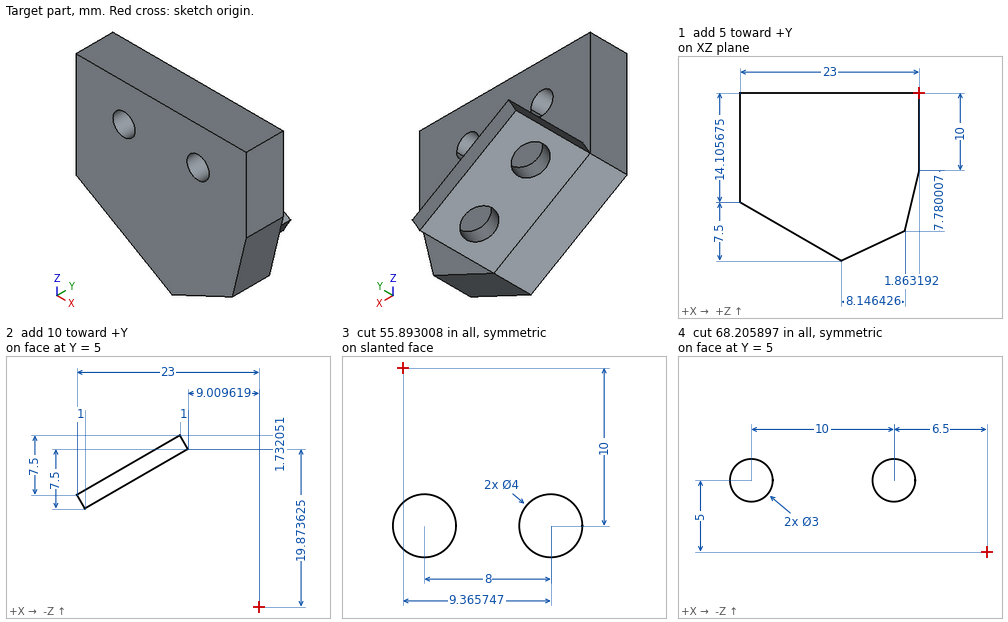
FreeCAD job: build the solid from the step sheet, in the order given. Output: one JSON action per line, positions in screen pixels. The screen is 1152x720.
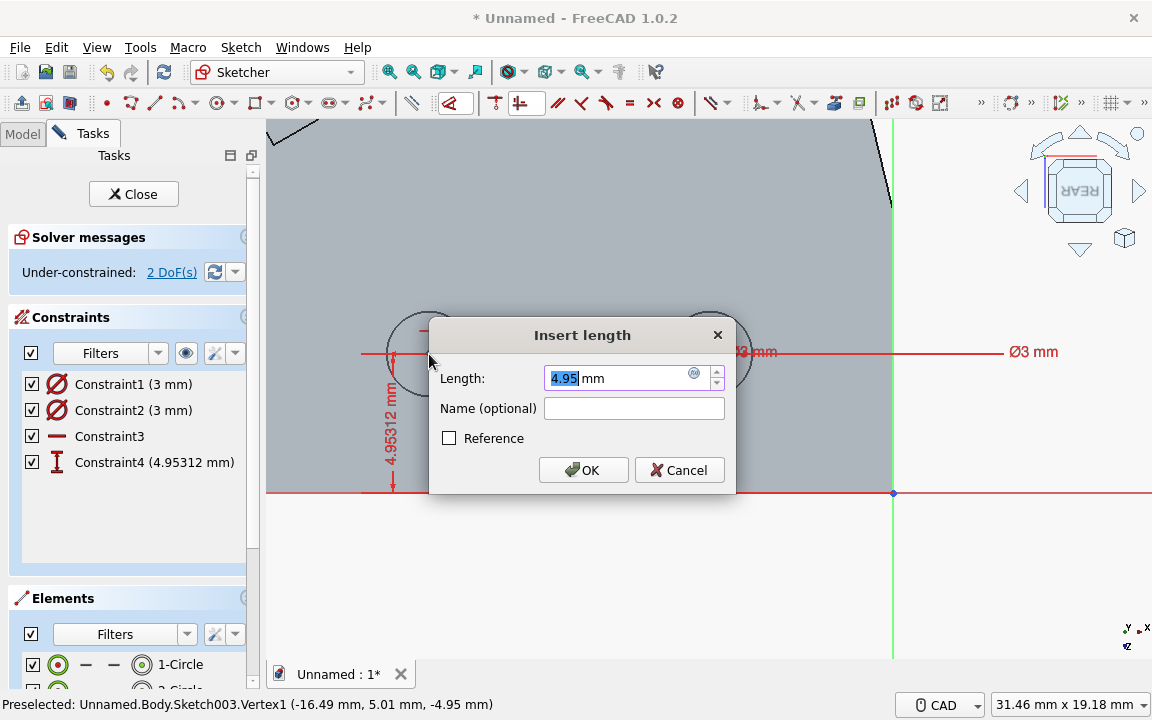
{"action": "type", "text": "5"}
{"action": "key", "text": "Return"}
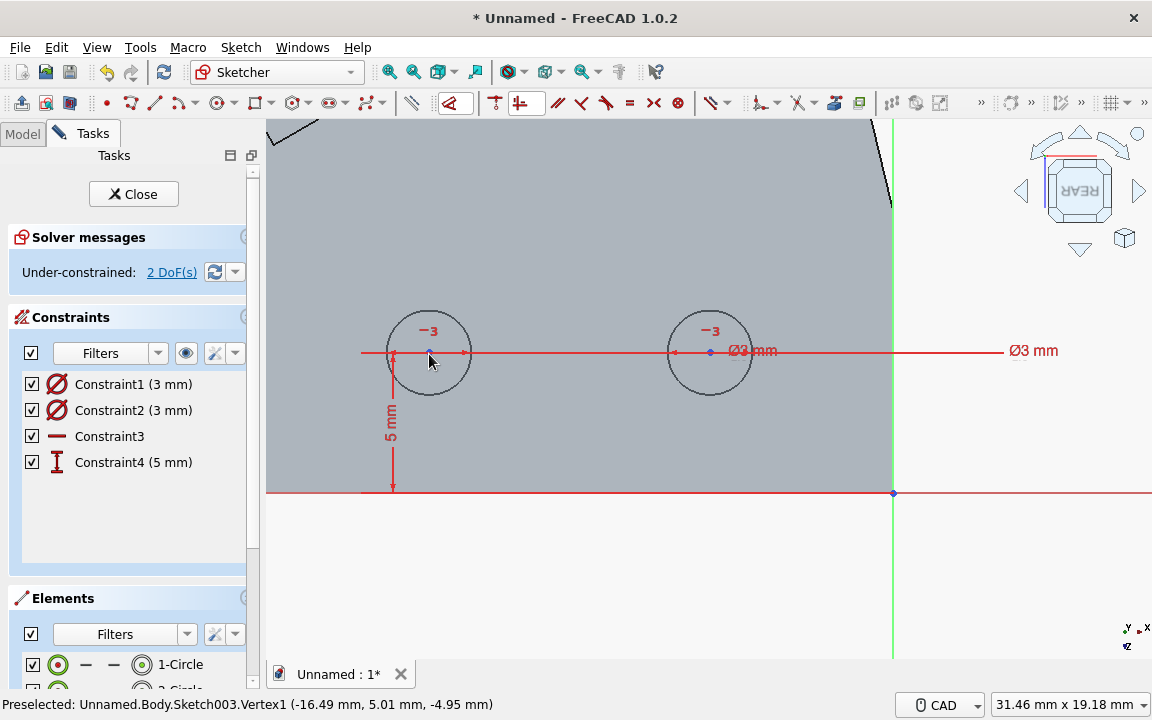
{"action": "left_click", "coordinate": [710, 353]}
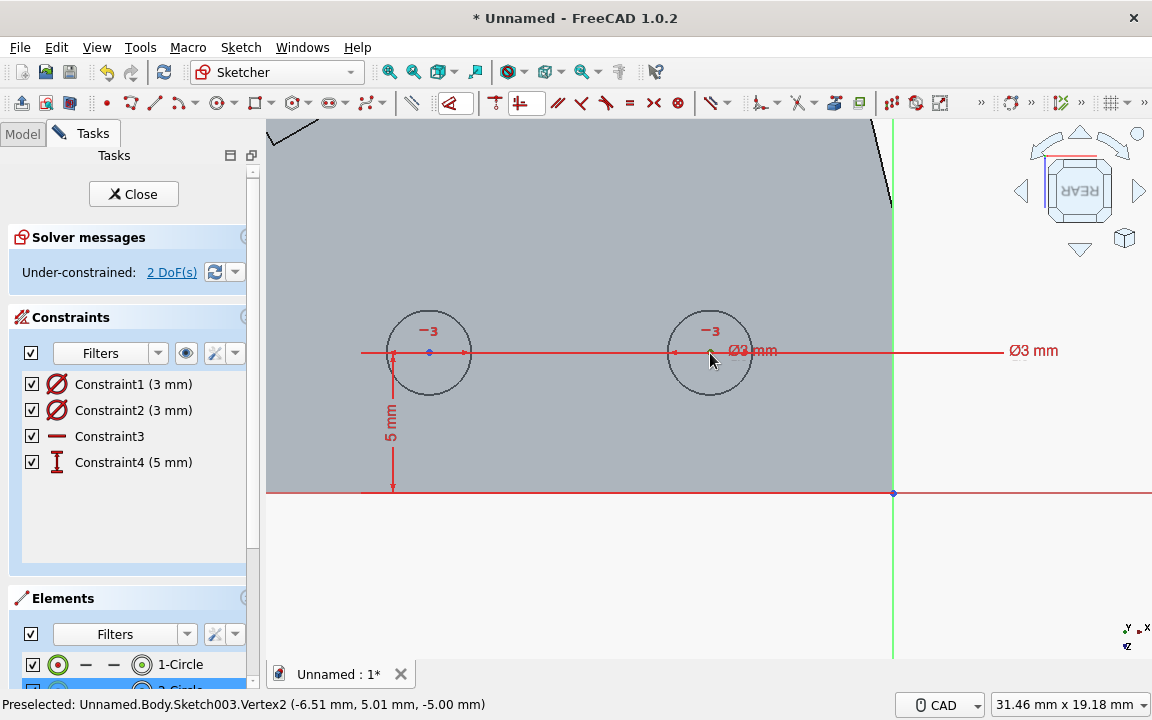
{"action": "left_click", "coordinate": [468, 104]}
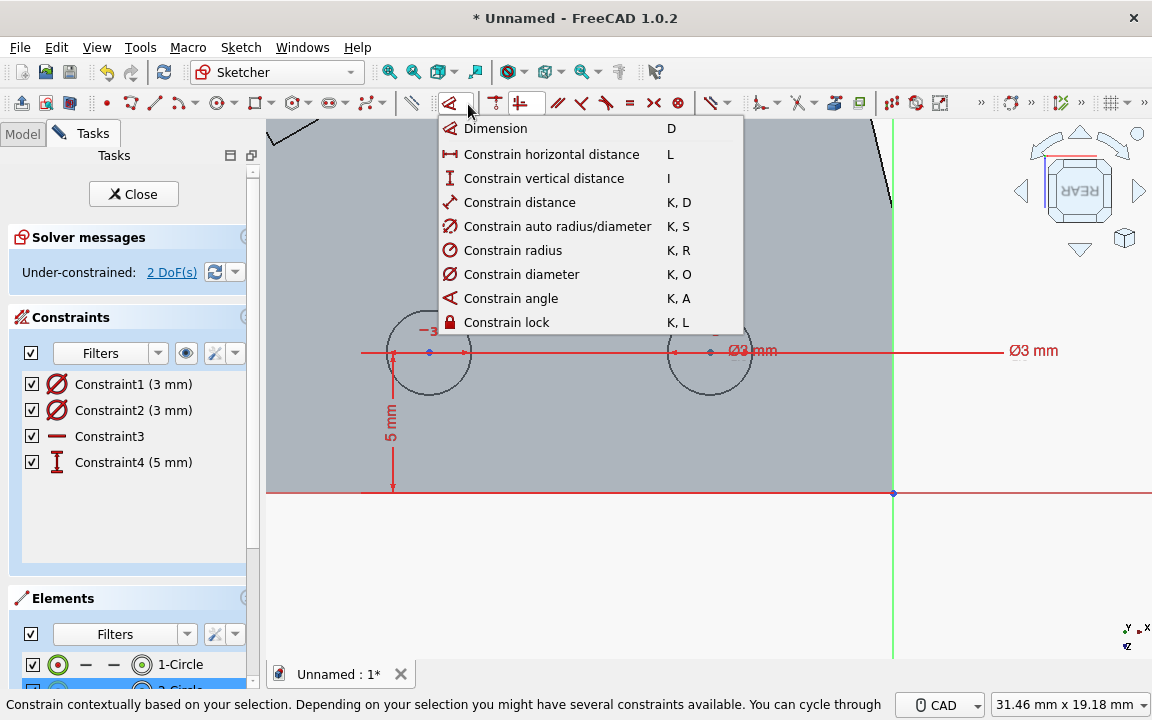
{"action": "left_click", "coordinate": [591, 154]}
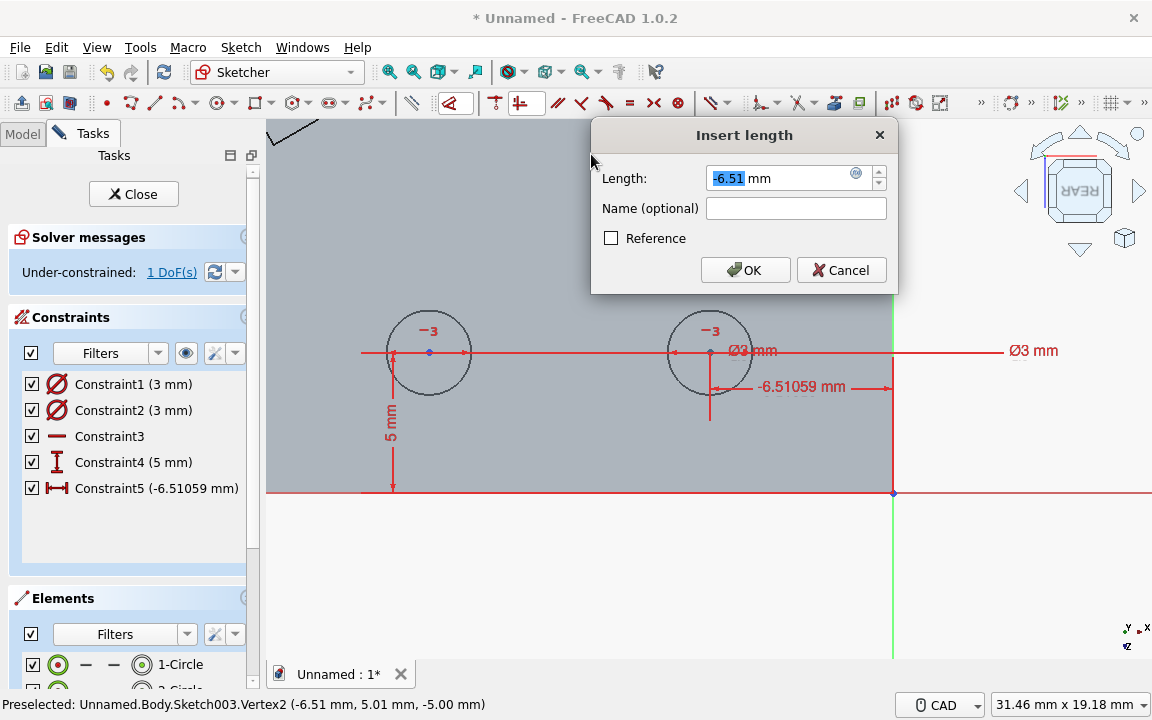
{"action": "type", "text": "-6.5"}
{"action": "key", "text": "Return"}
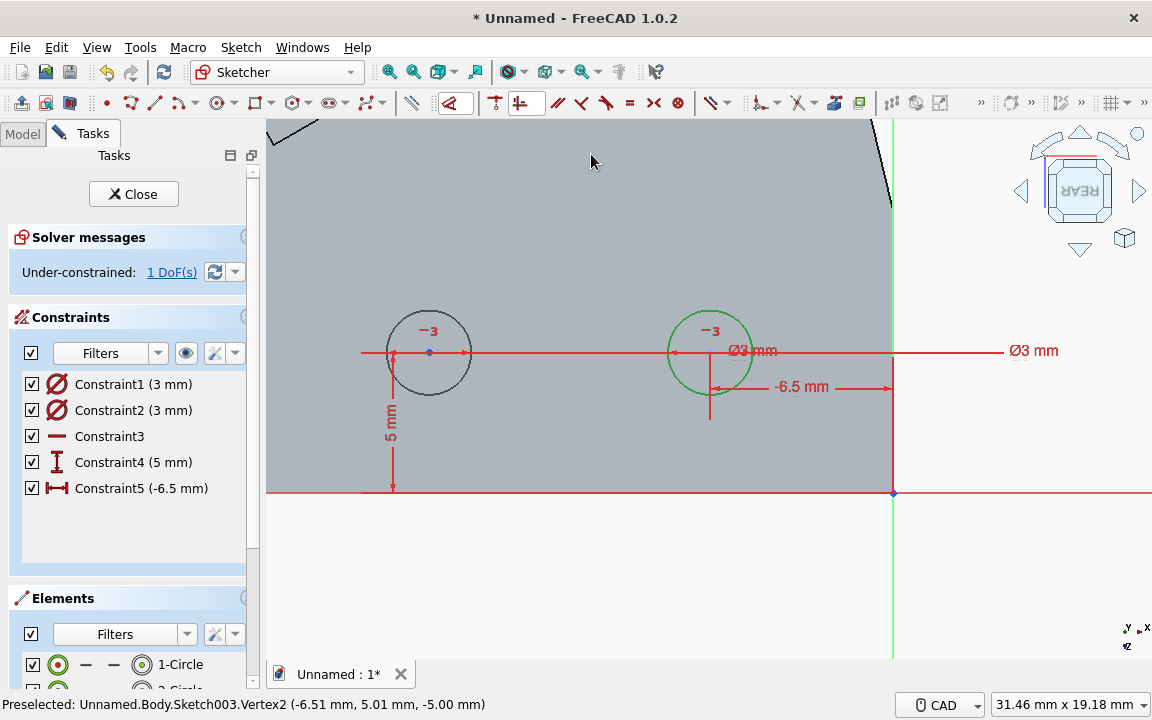
{"action": "left_click", "coordinate": [429, 353]}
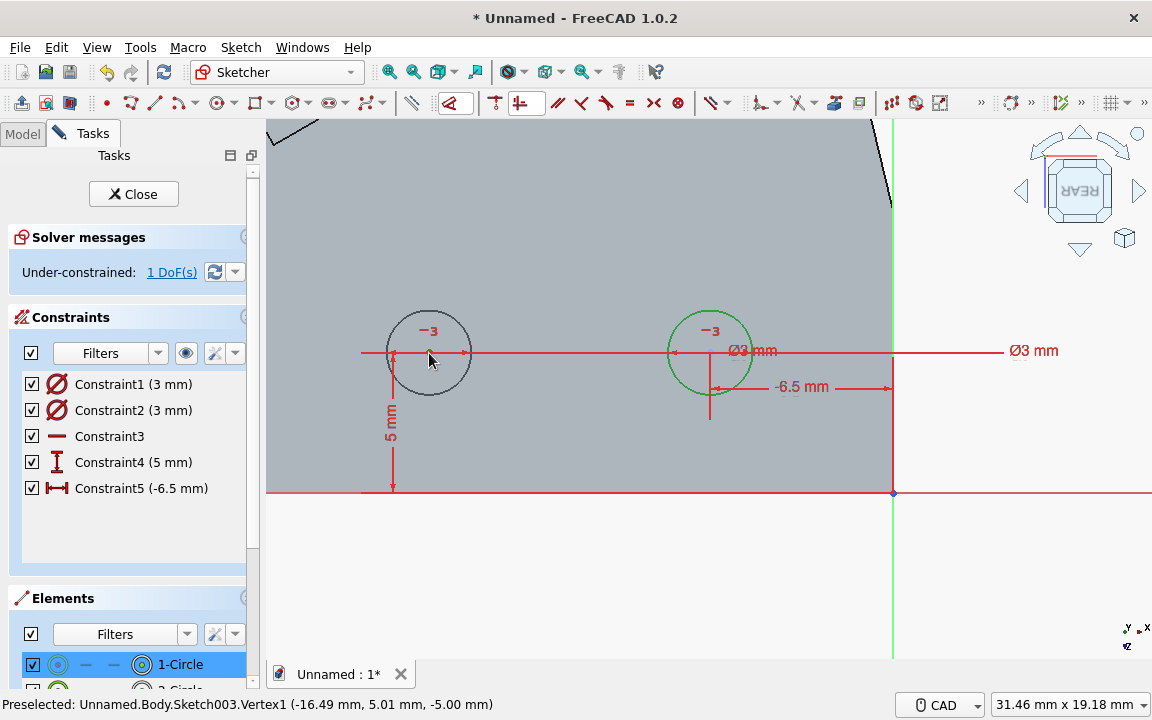
{"action": "left_click", "coordinate": [710, 353]}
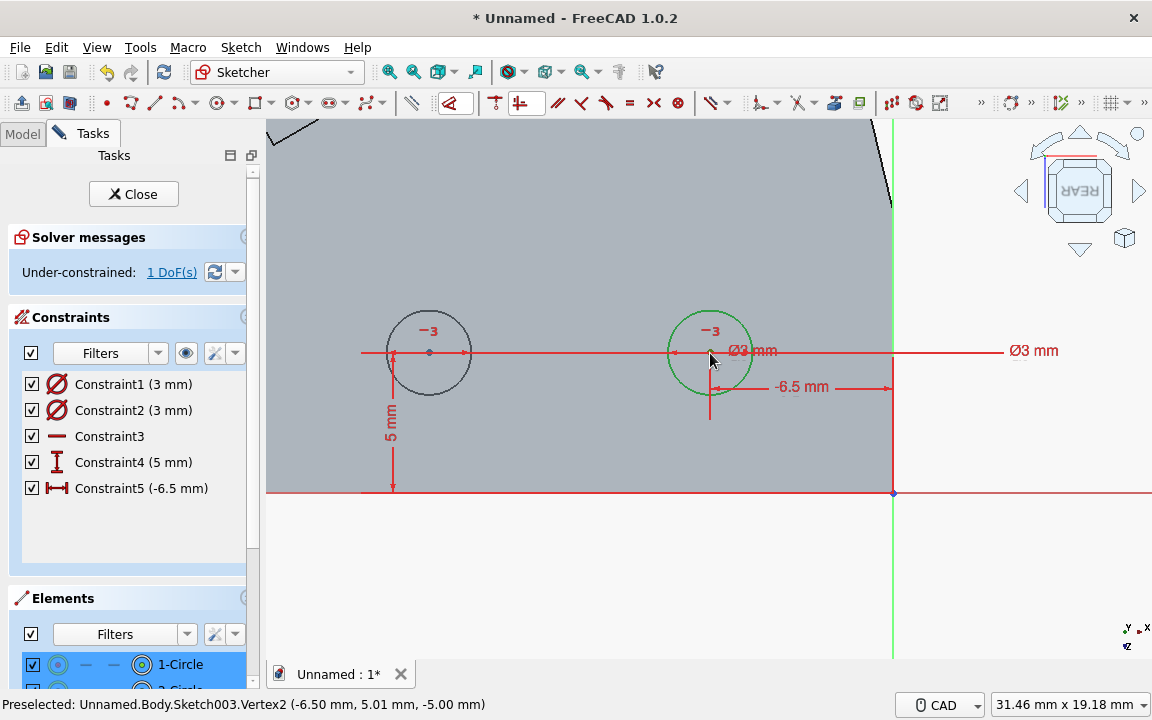
{"action": "key", "text": "l"}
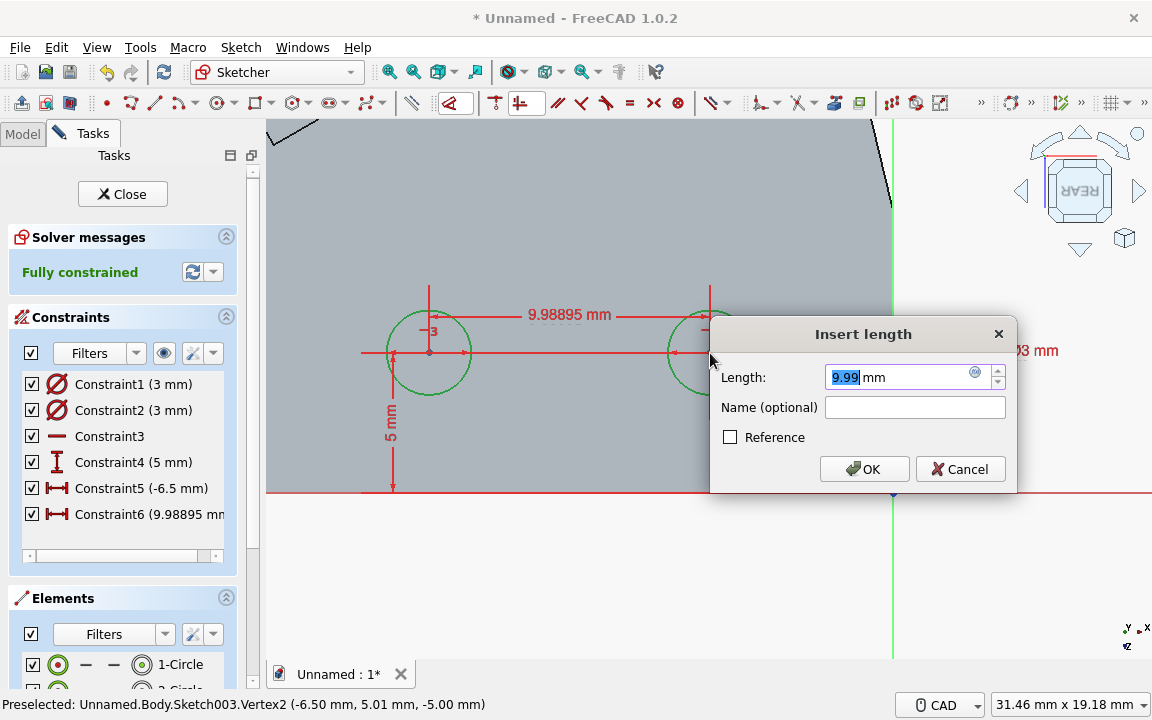
{"action": "type", "text": "10"}
{"action": "key", "text": "Return"}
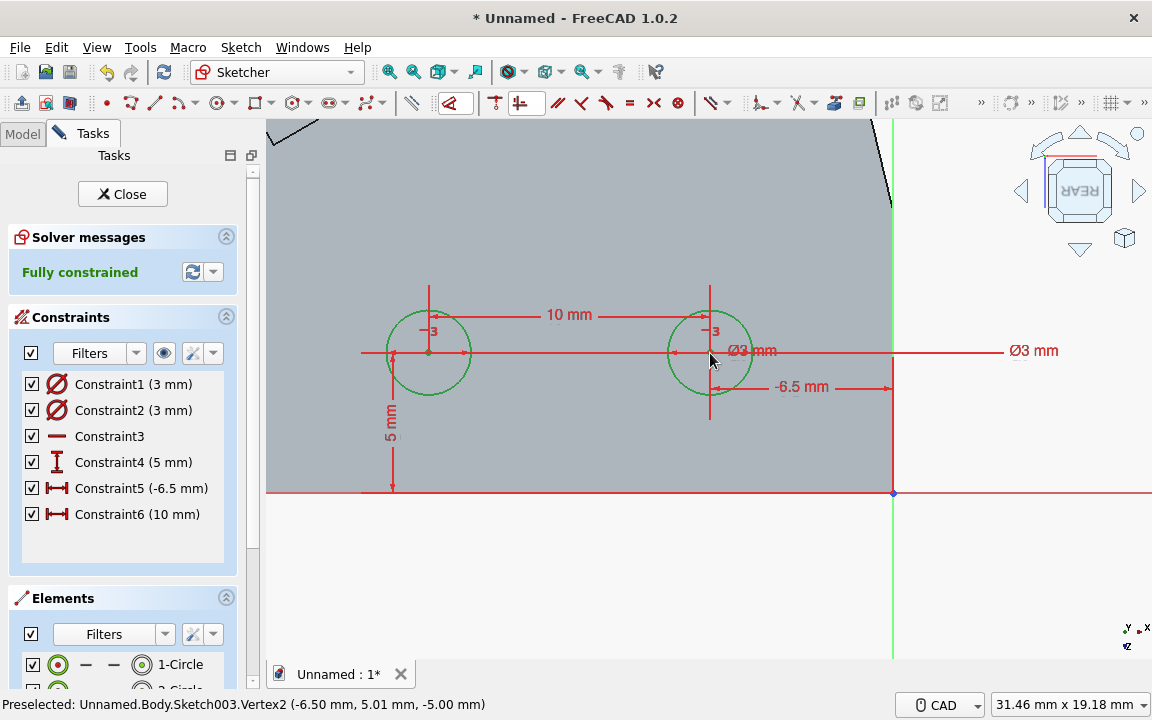
{"action": "left_click", "coordinate": [123, 194]}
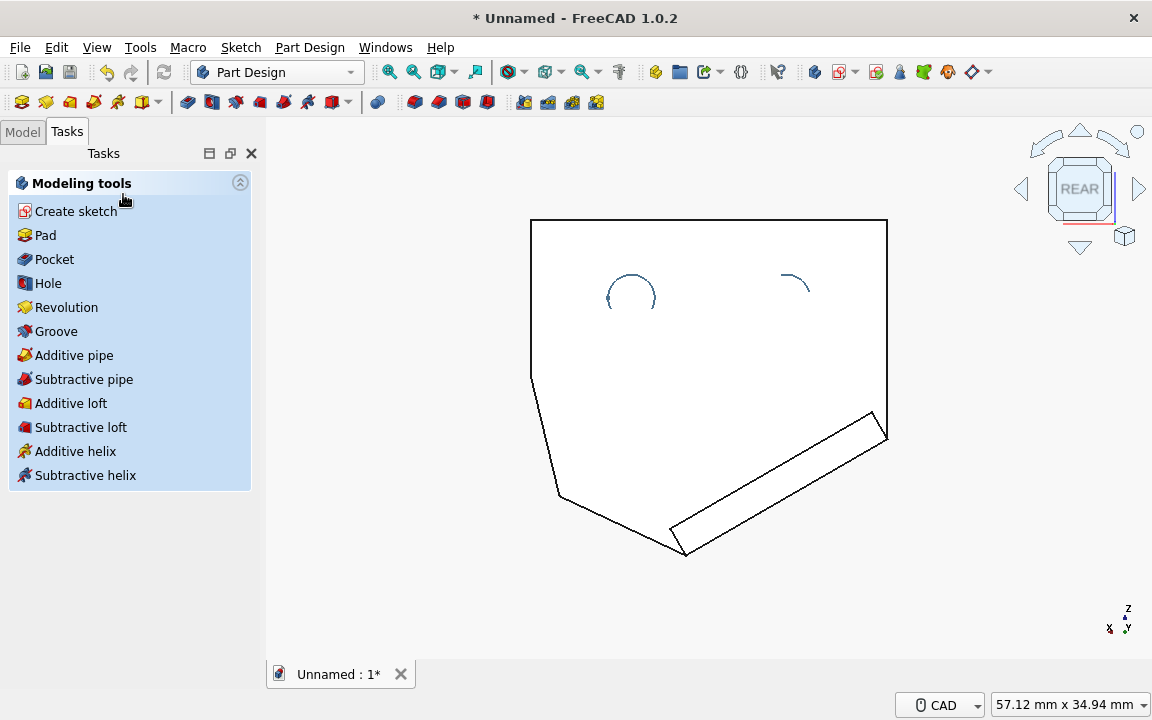
{"action": "left_click", "coordinate": [188, 102]}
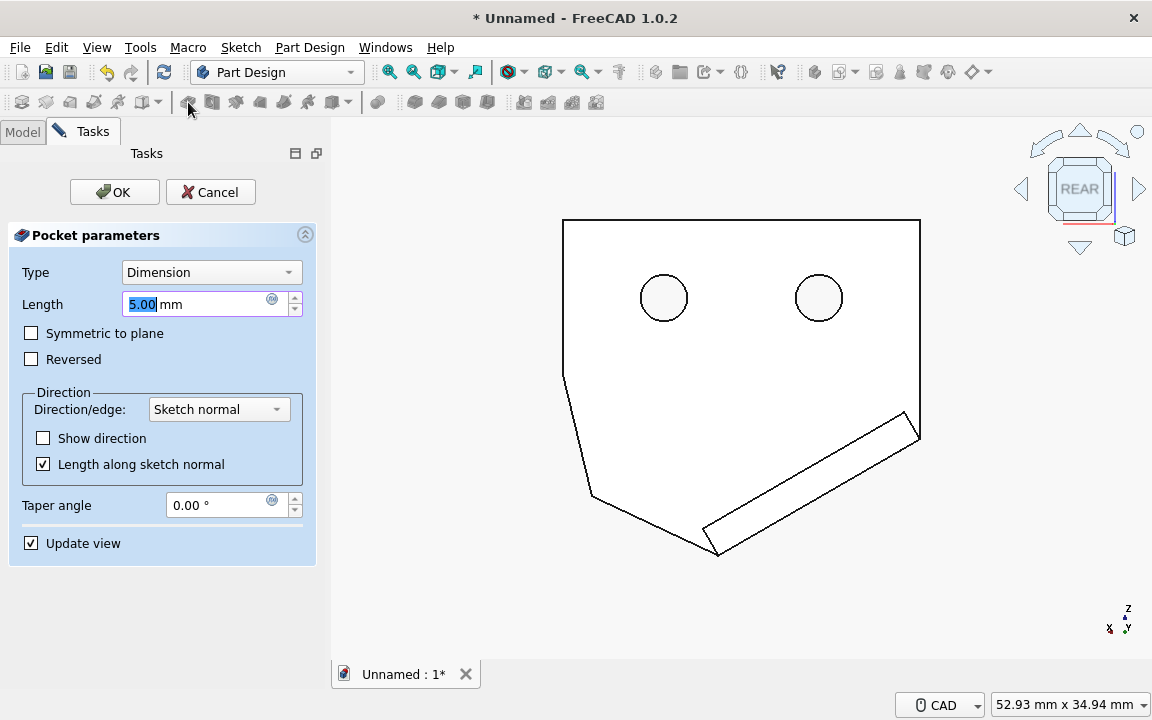
{"action": "type", "text": "68.205897"}
{"action": "key", "text": "Tab"}